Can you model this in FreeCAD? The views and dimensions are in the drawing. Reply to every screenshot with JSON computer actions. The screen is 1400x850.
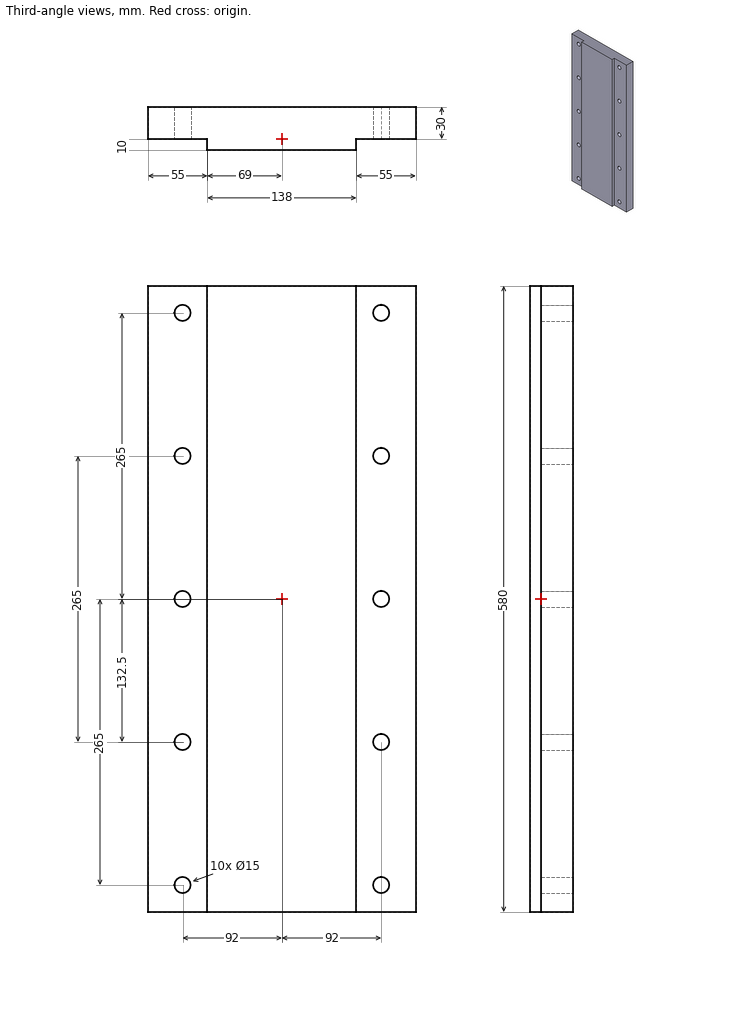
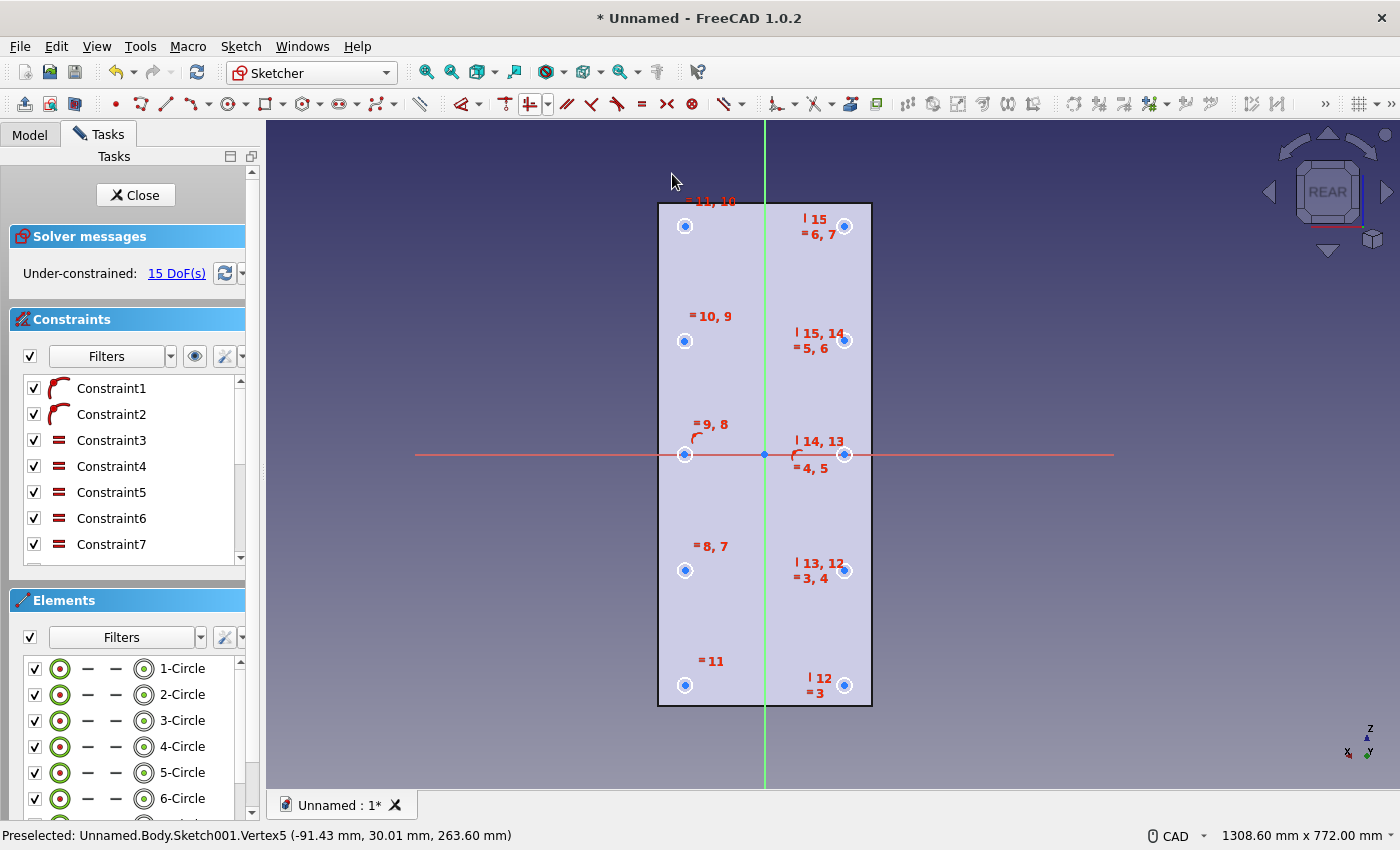
{"action": "left_click", "coordinate": [844, 571]}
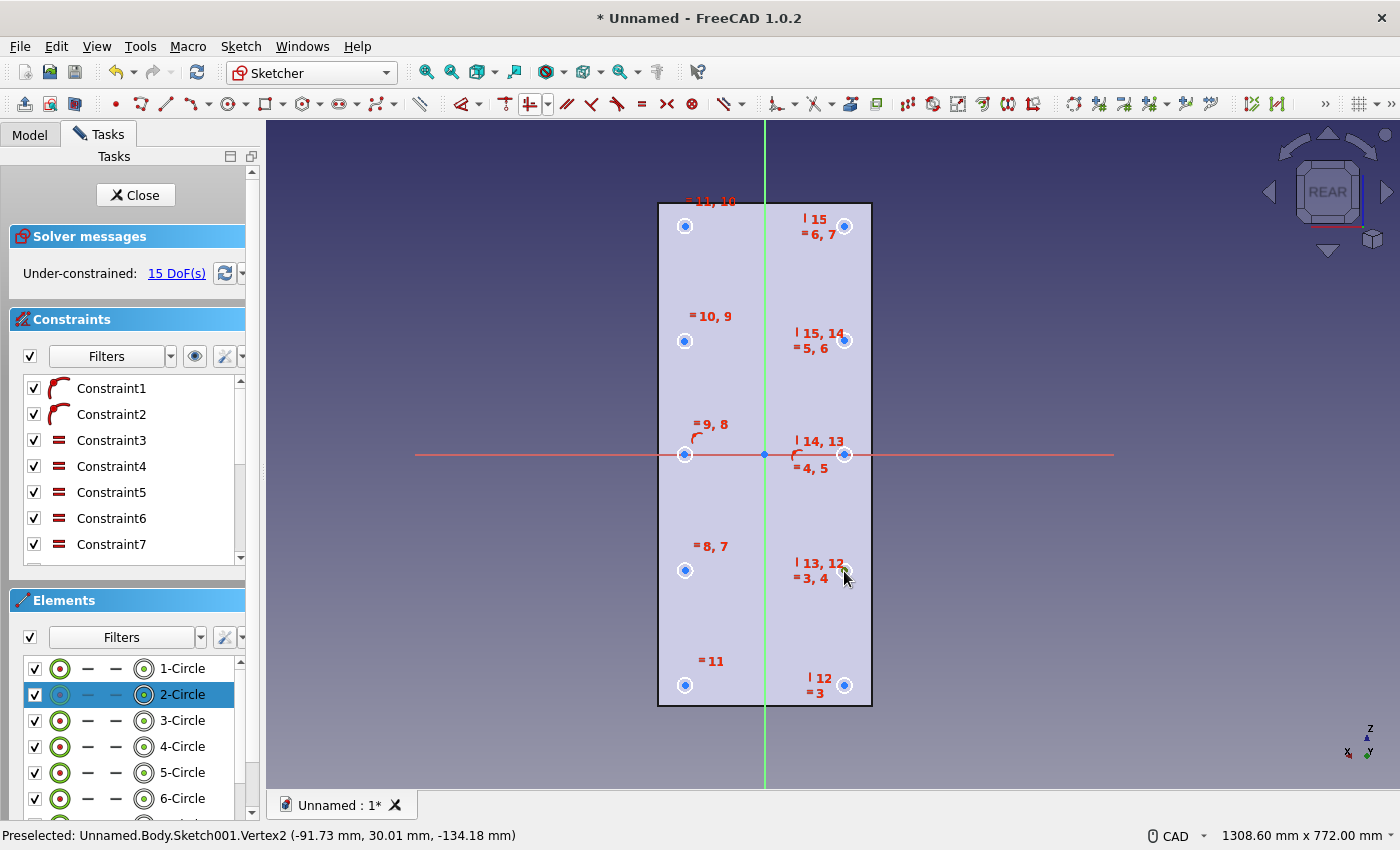
{"action": "left_click", "coordinate": [685, 571]}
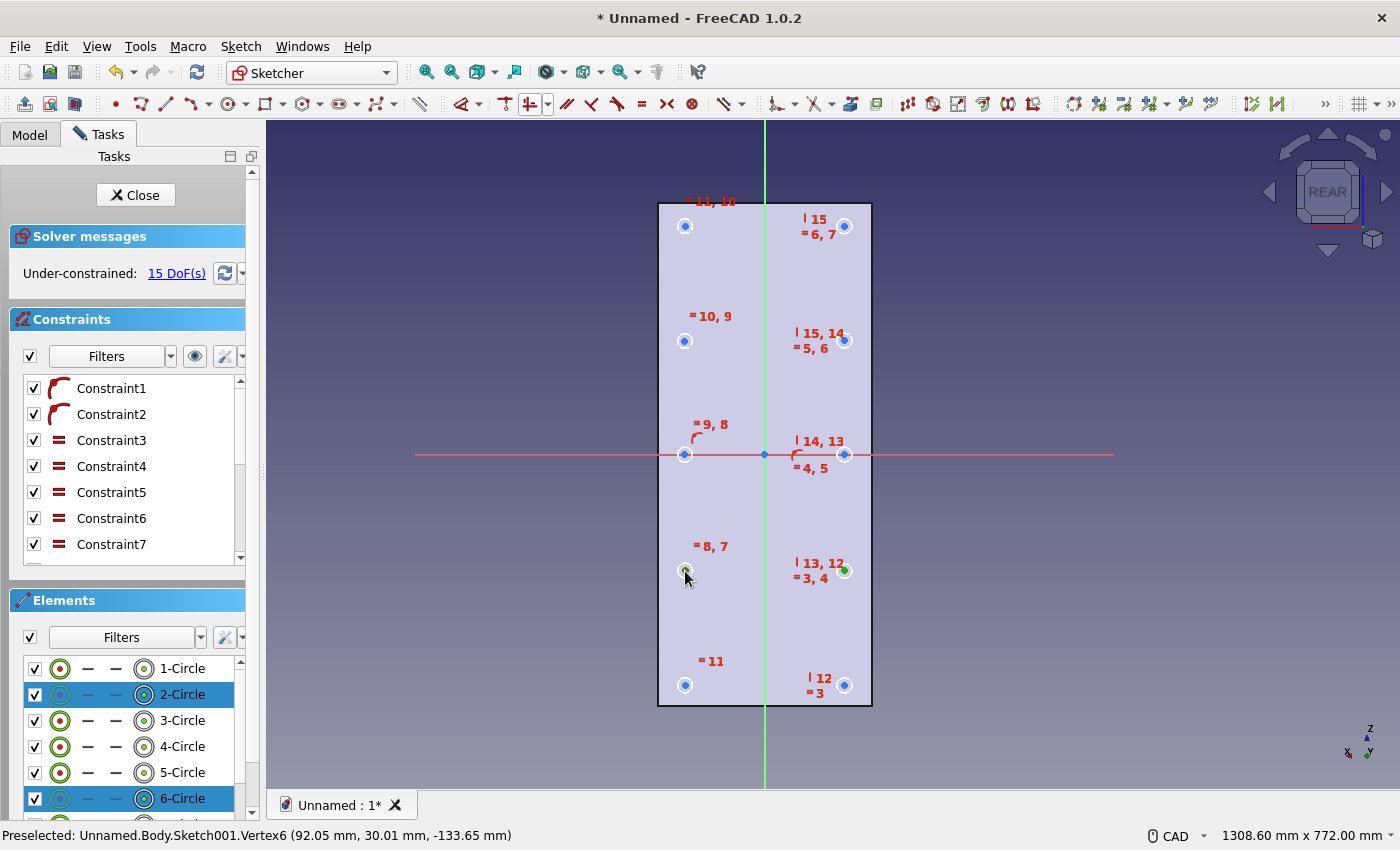
{"action": "key", "text": "h"}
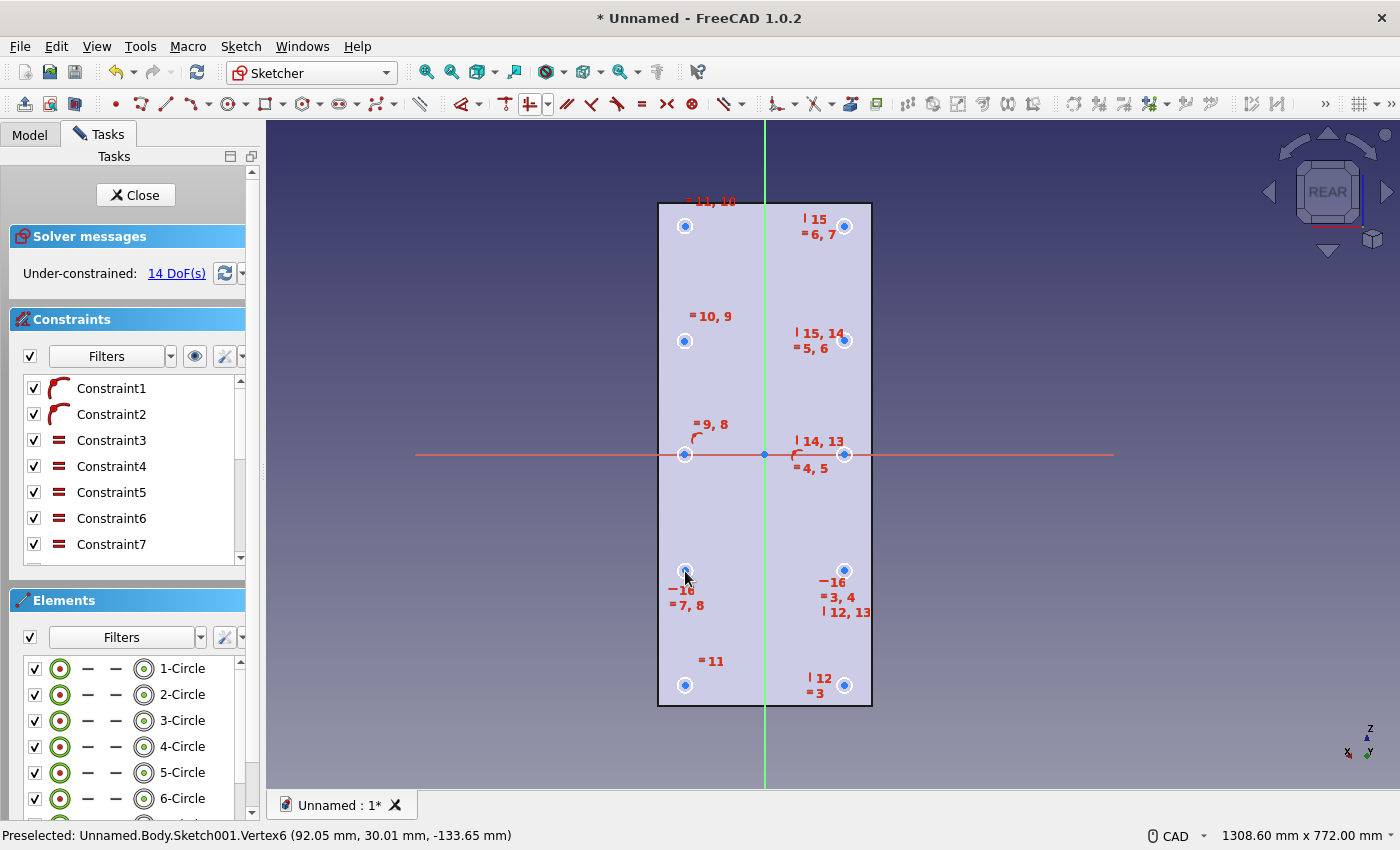
{"action": "left_click", "coordinate": [685, 571]}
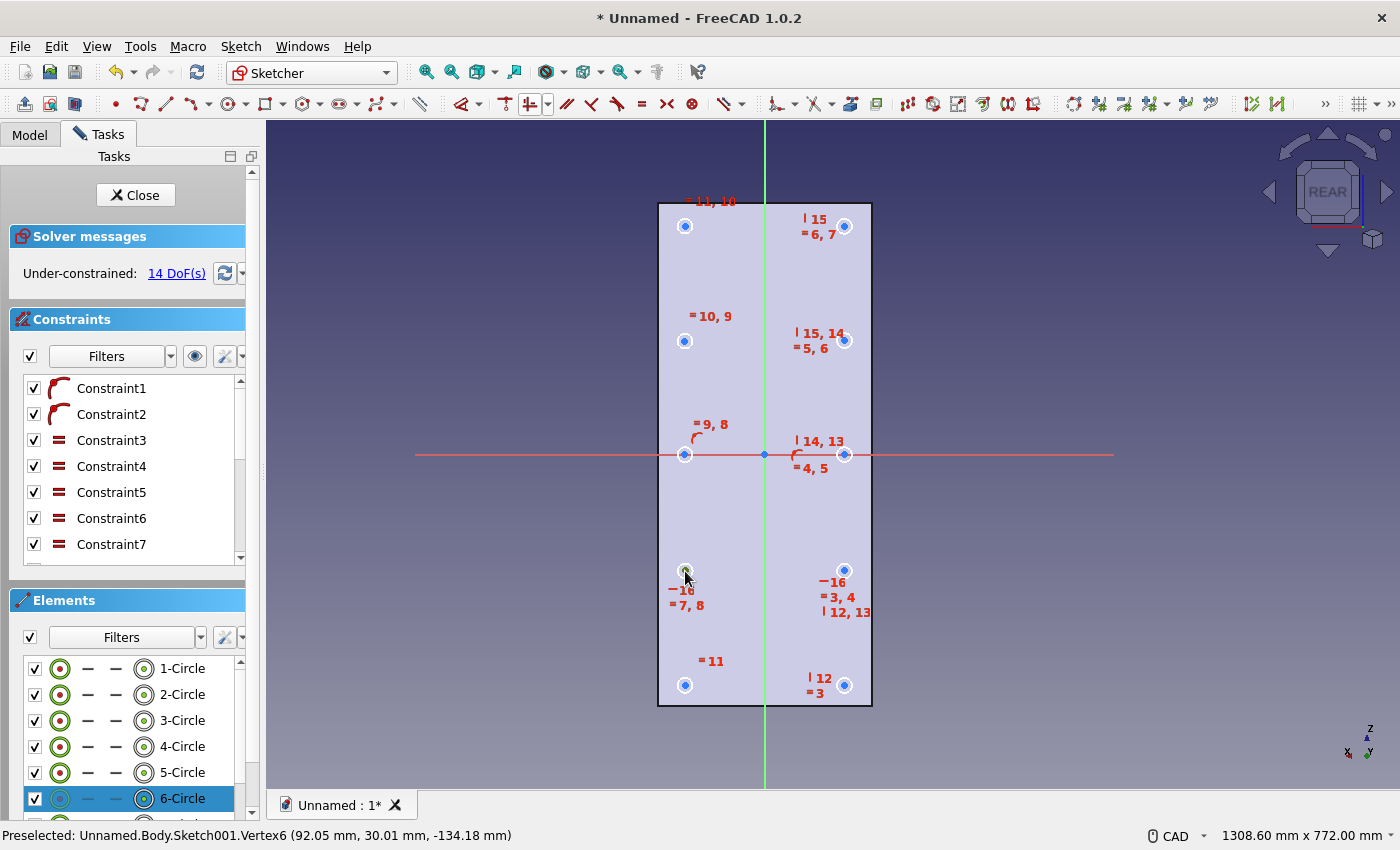
{"action": "left_click", "coordinate": [685, 455]}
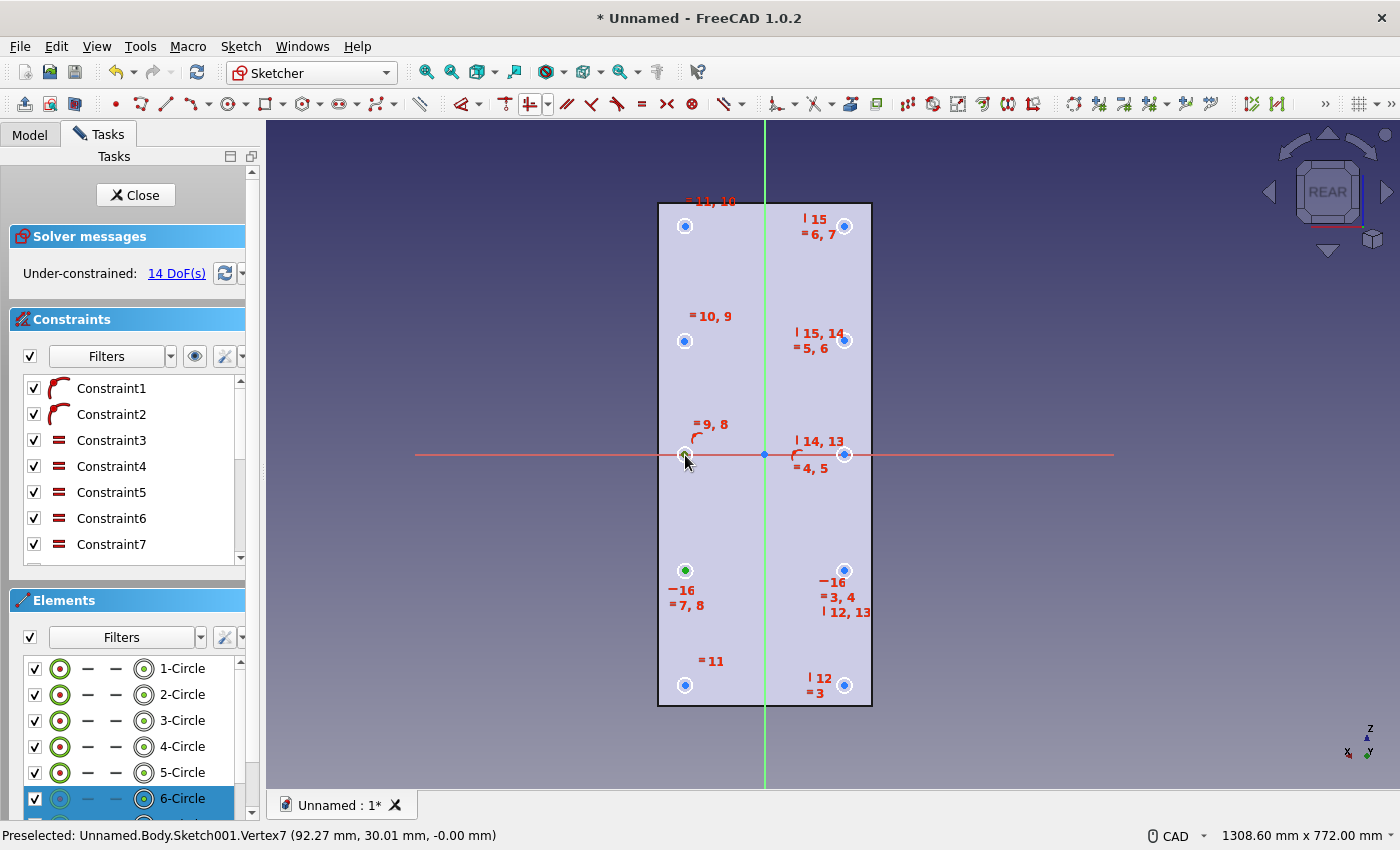
{"action": "key", "text": "v"}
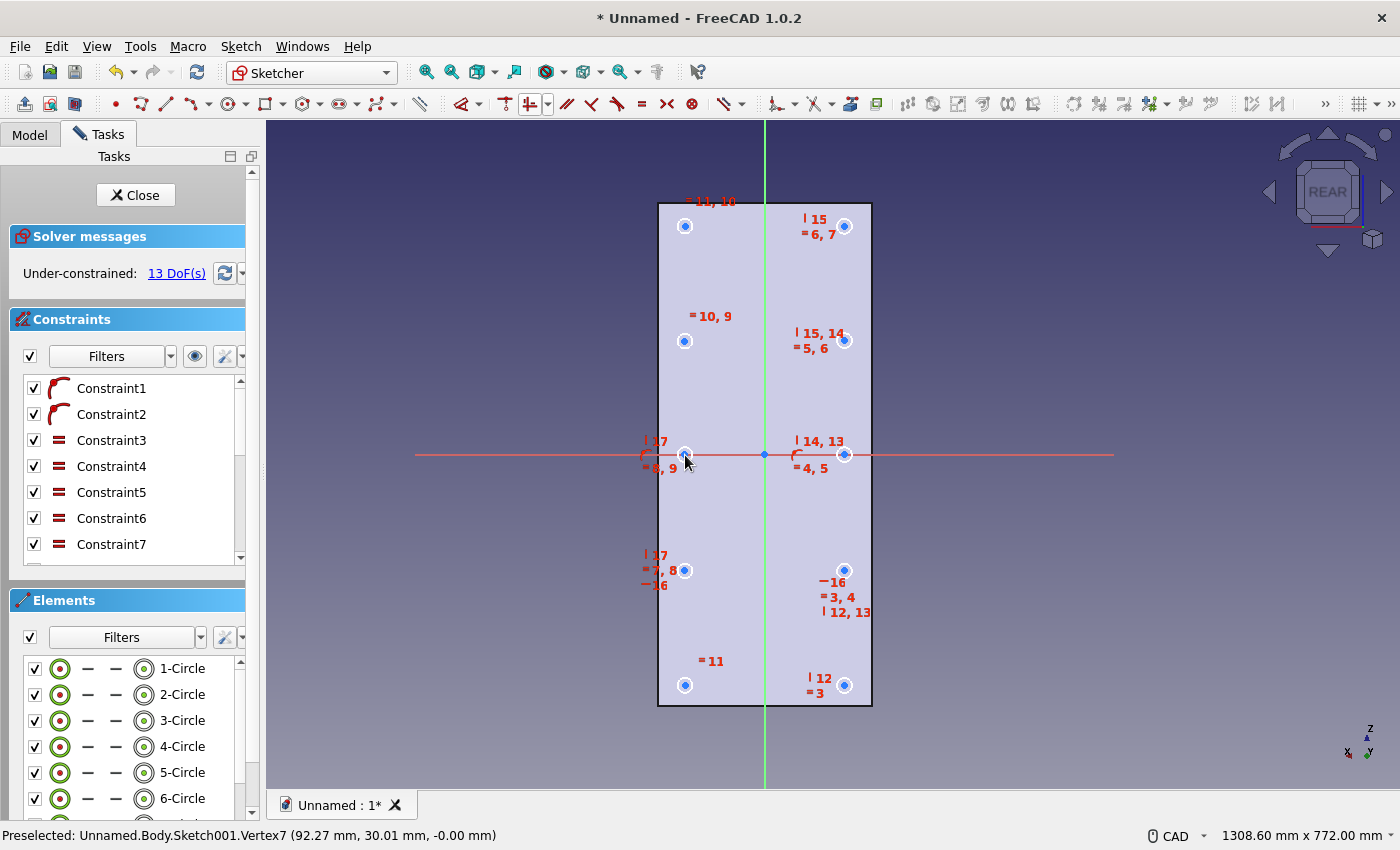
{"action": "left_click", "coordinate": [685, 455]}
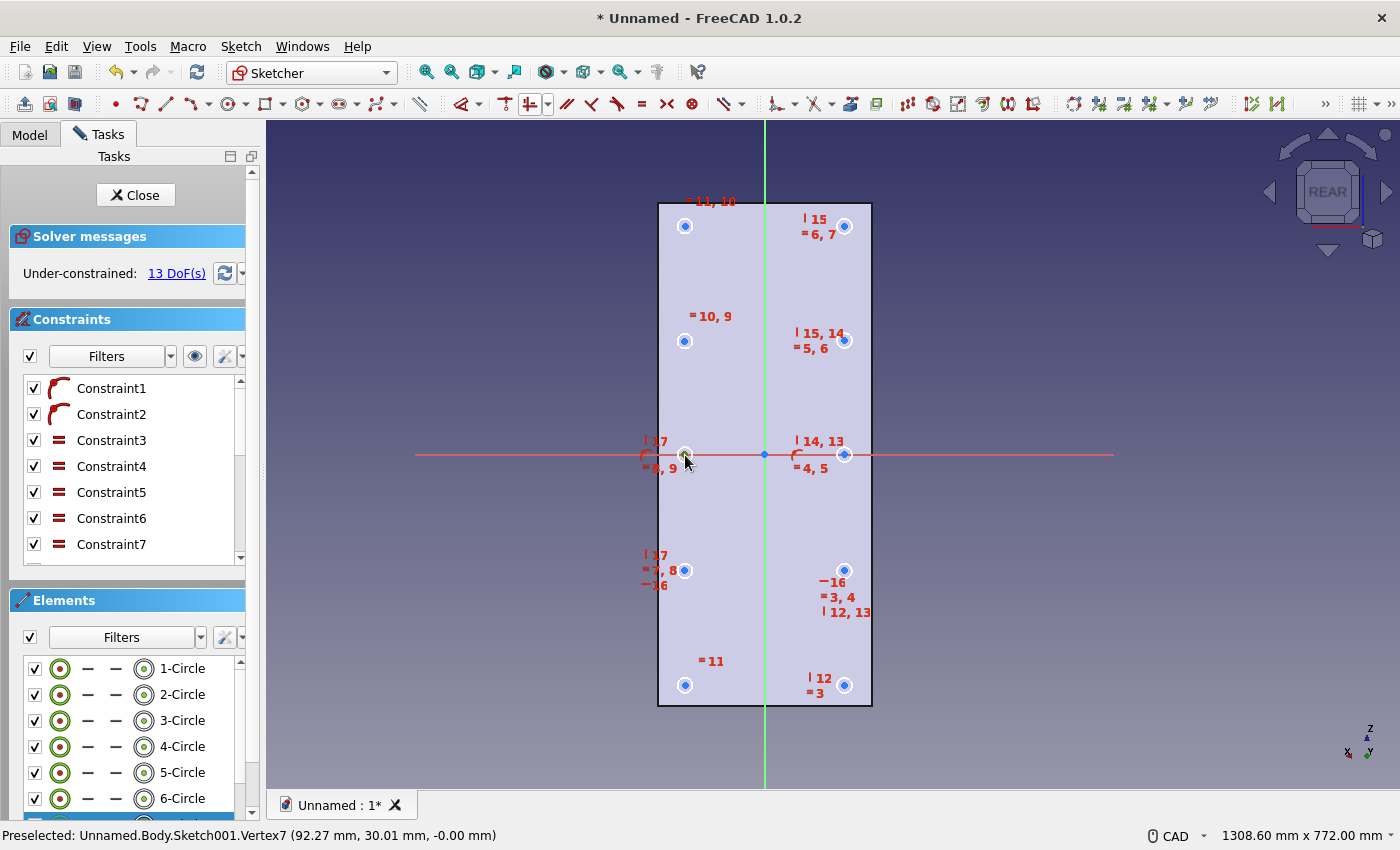
{"action": "left_click", "coordinate": [685, 341]}